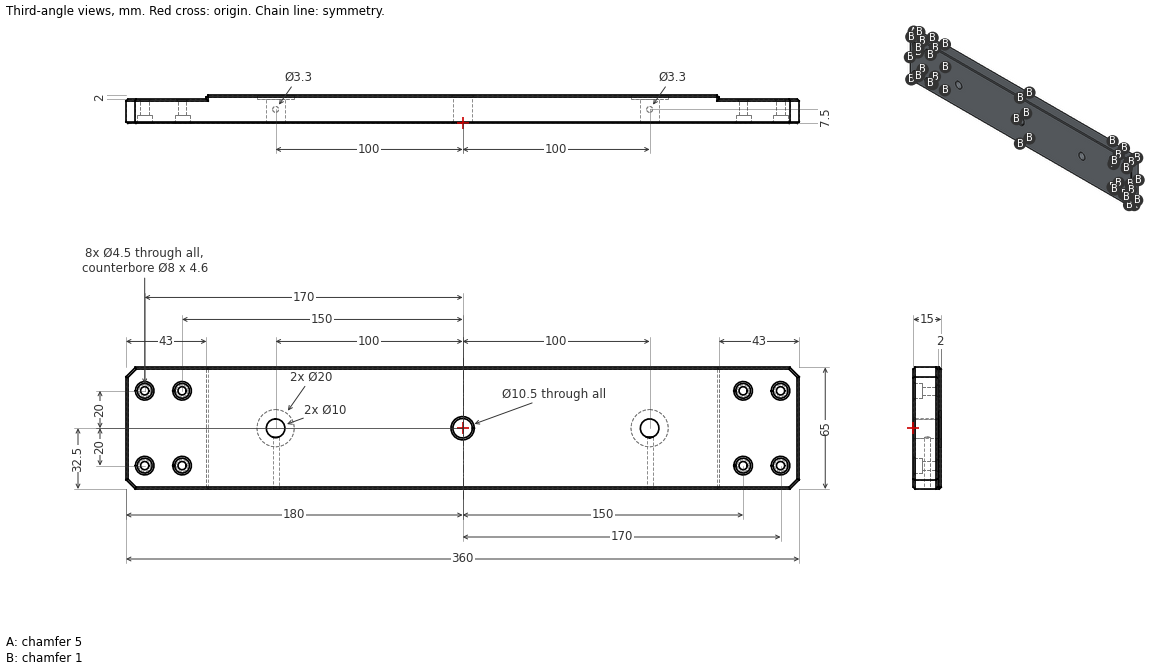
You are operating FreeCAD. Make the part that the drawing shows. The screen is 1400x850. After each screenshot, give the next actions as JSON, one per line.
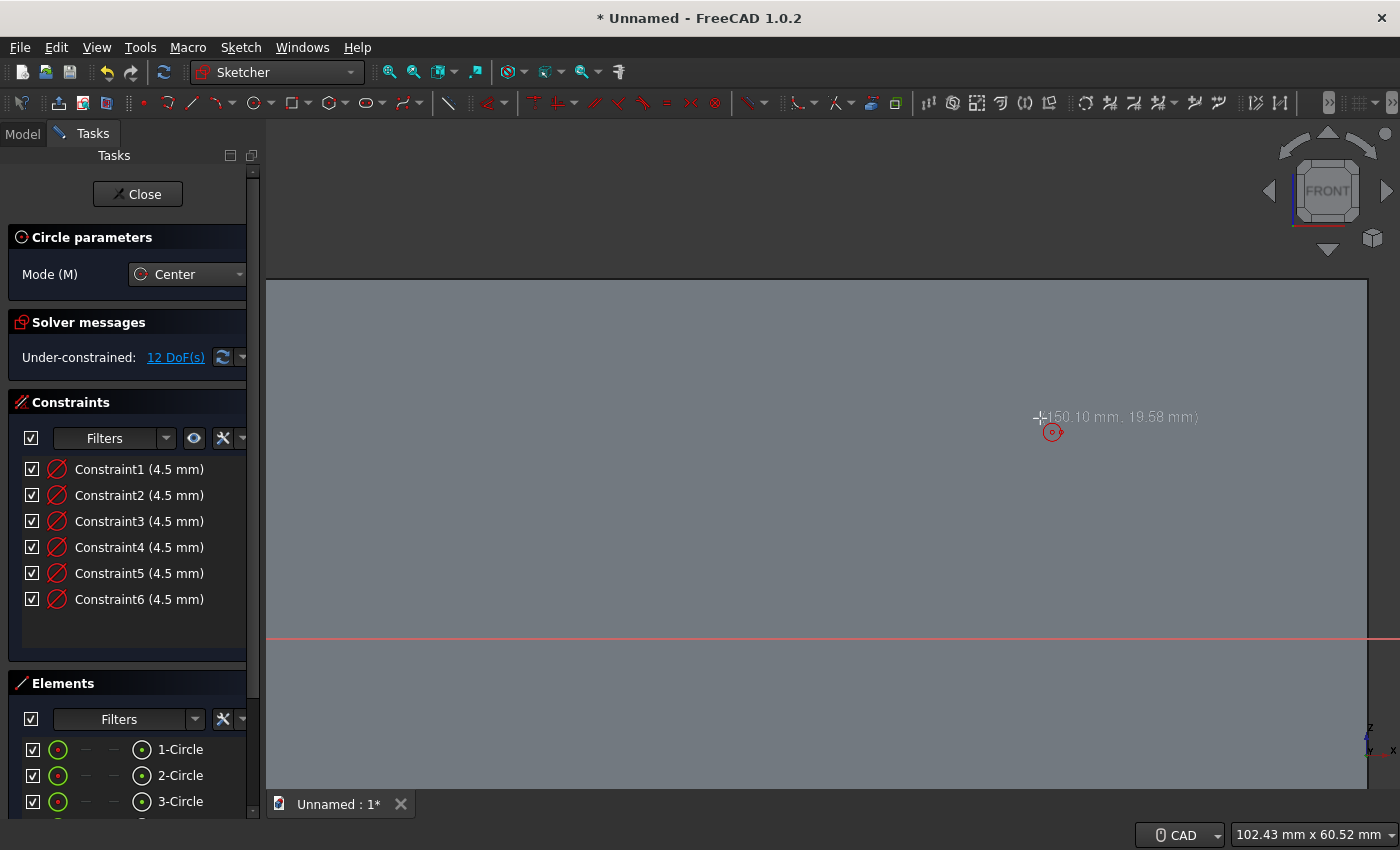
{"action": "scroll", "coordinate": [1040, 417], "scroll_direction": "down", "scroll_amount": 9}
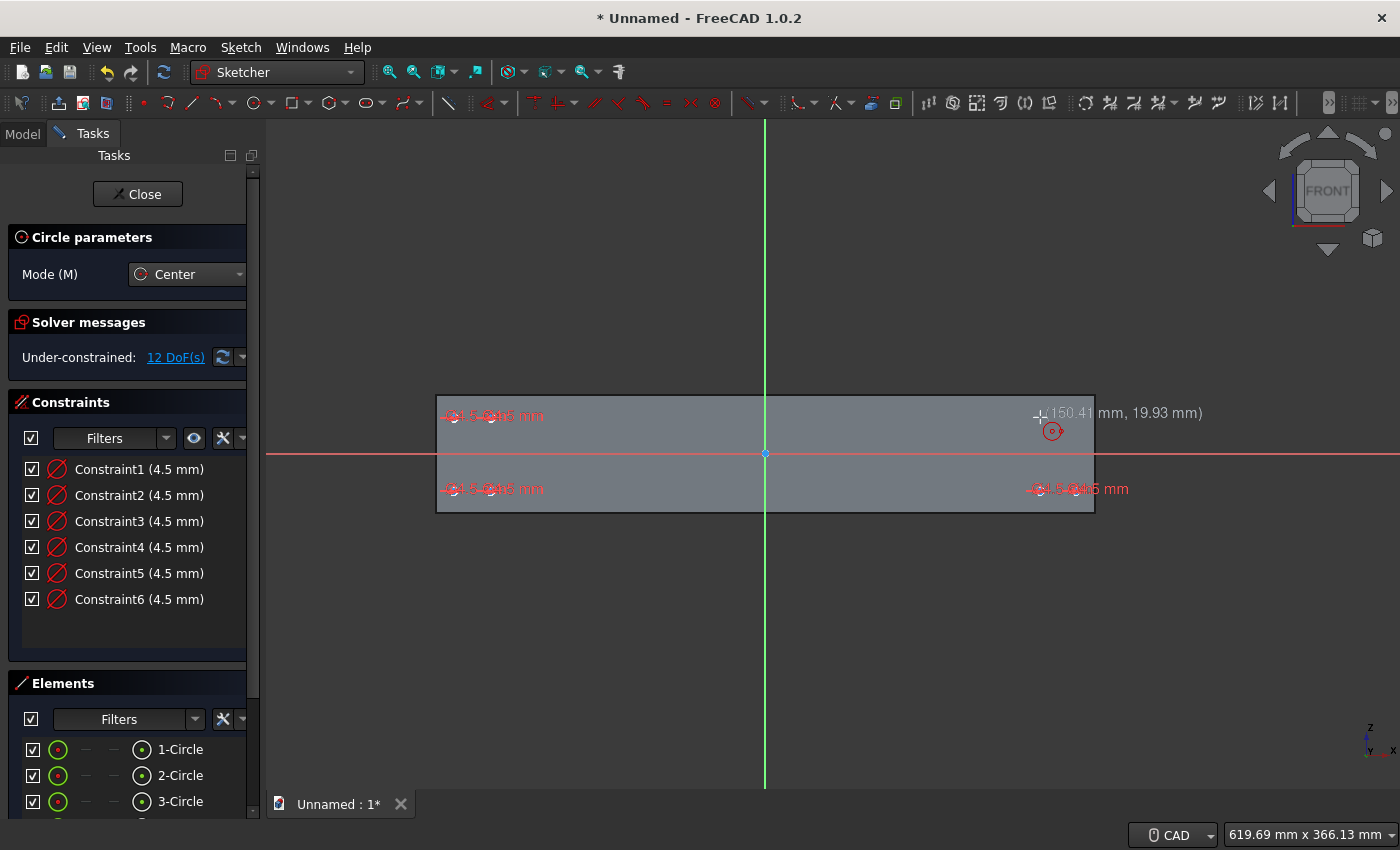
{"action": "left_click", "coordinate": [1040, 417]}
{"action": "mouse_move", "coordinate": [1043, 414]}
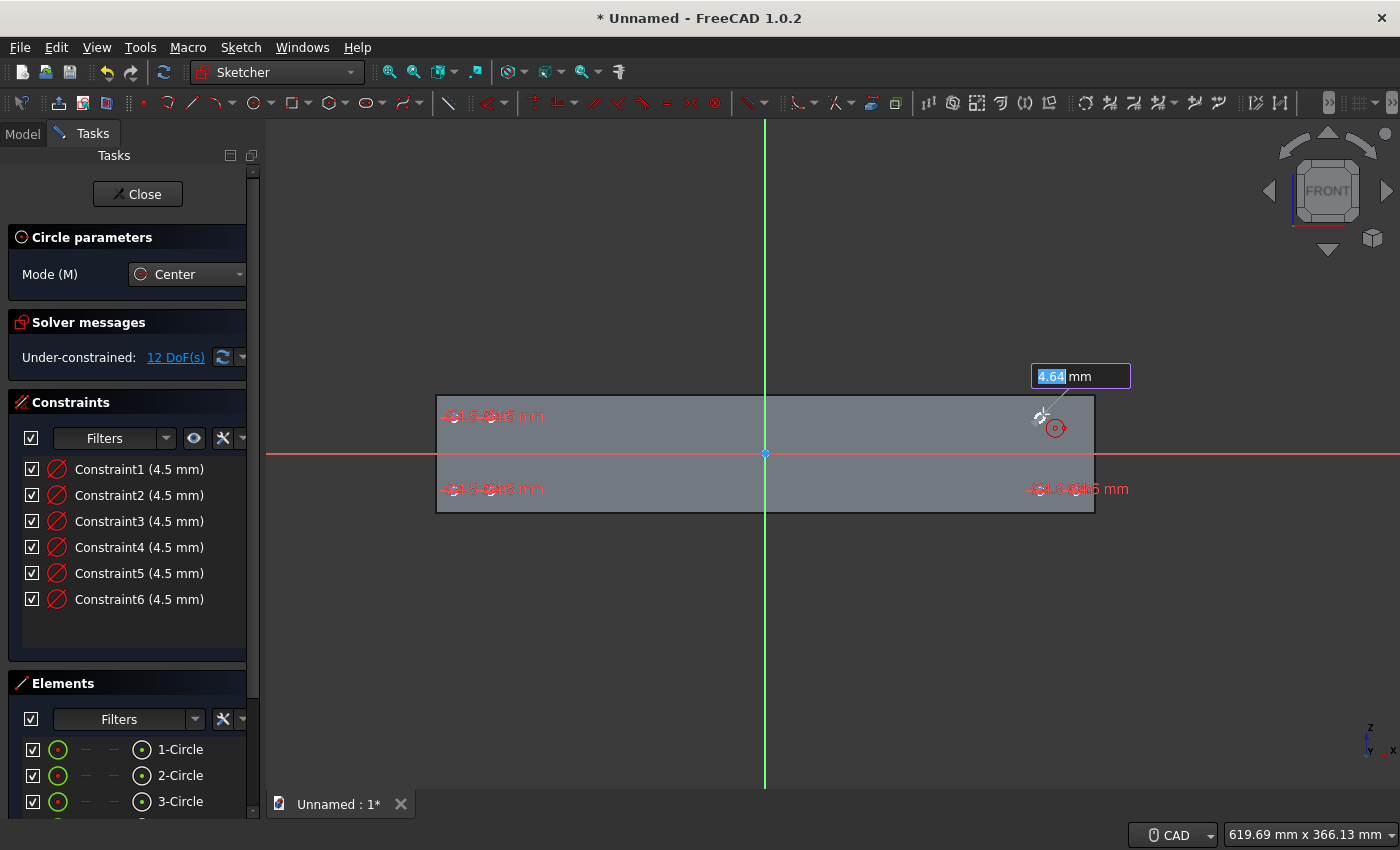
{"action": "type", "text": "4.5"}
{"action": "key", "text": "Return"}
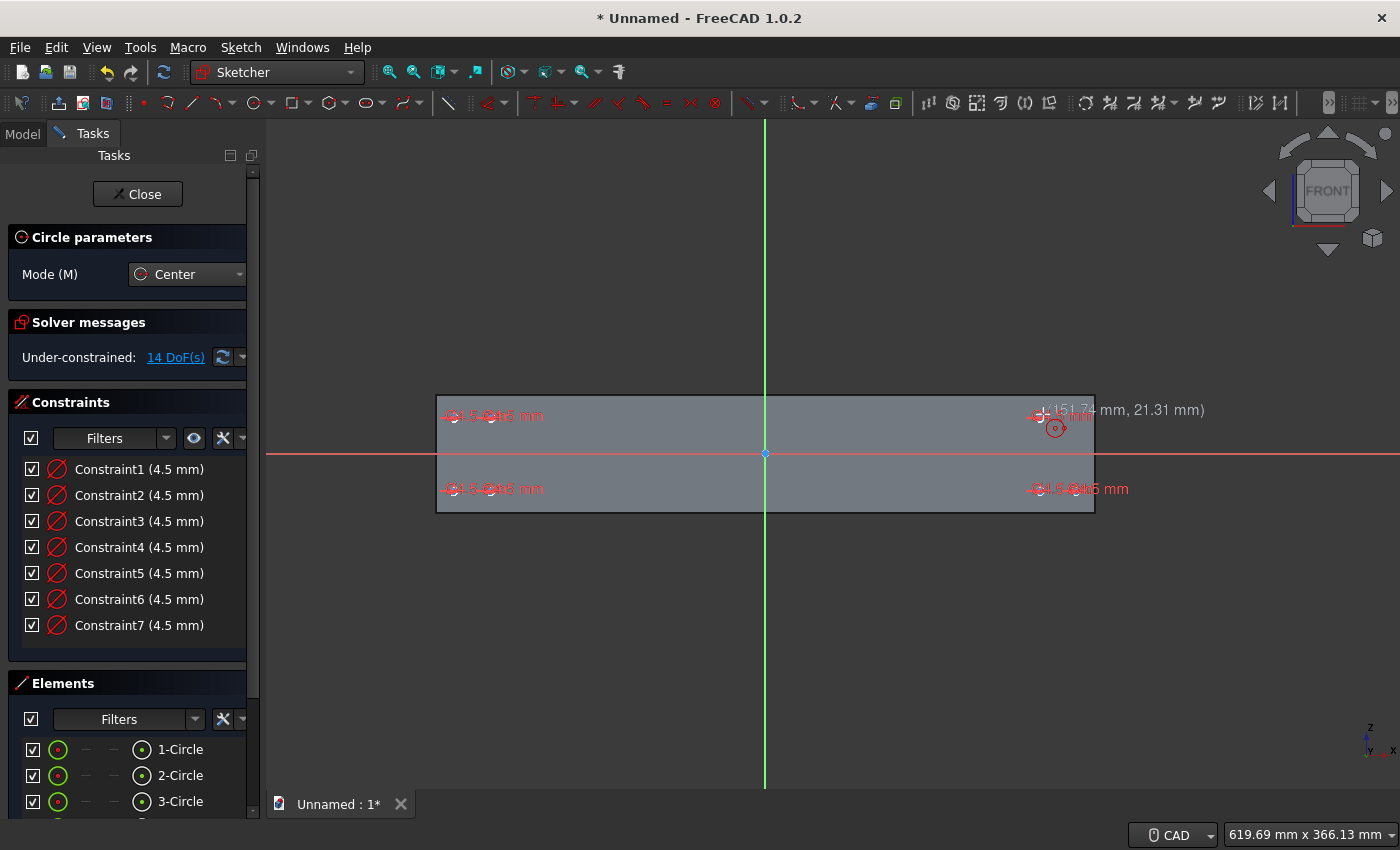
{"action": "scroll", "coordinate": [1076, 417], "scroll_direction": "up", "scroll_amount": 9}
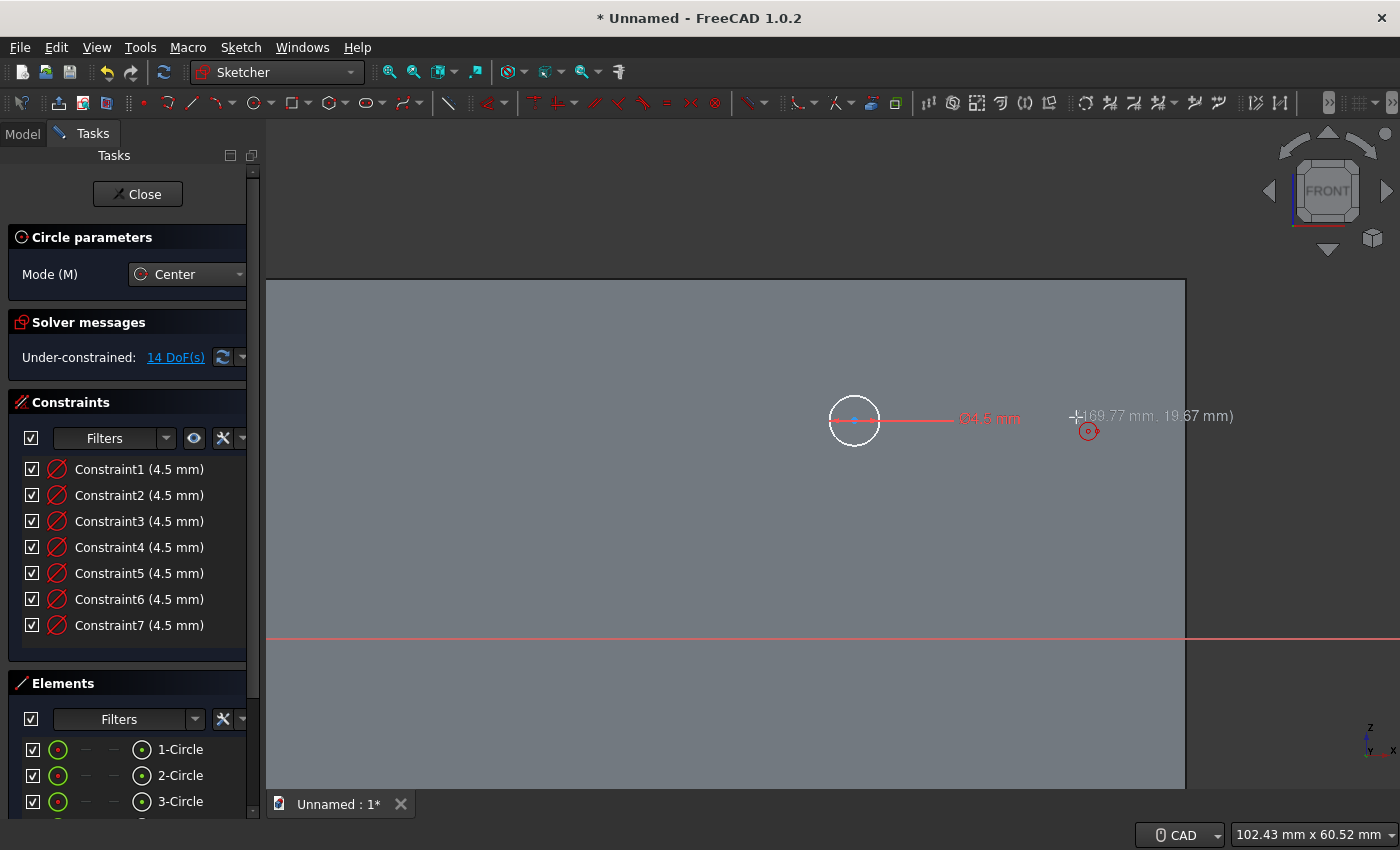
{"action": "scroll", "coordinate": [1076, 417], "scroll_direction": "down", "scroll_amount": 9}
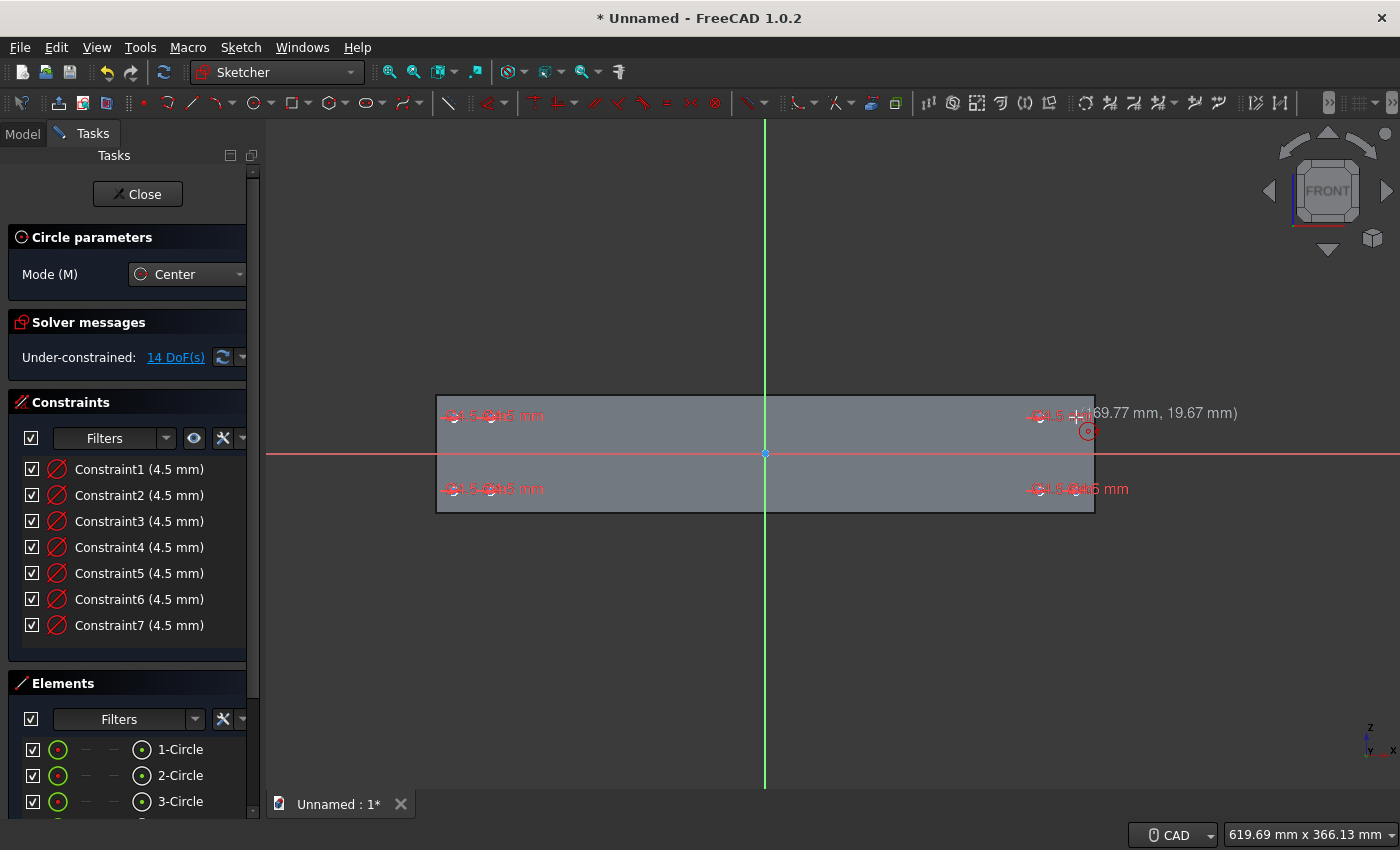
{"action": "left_click", "coordinate": [1076, 417]}
{"action": "mouse_move", "coordinate": [1079, 414]}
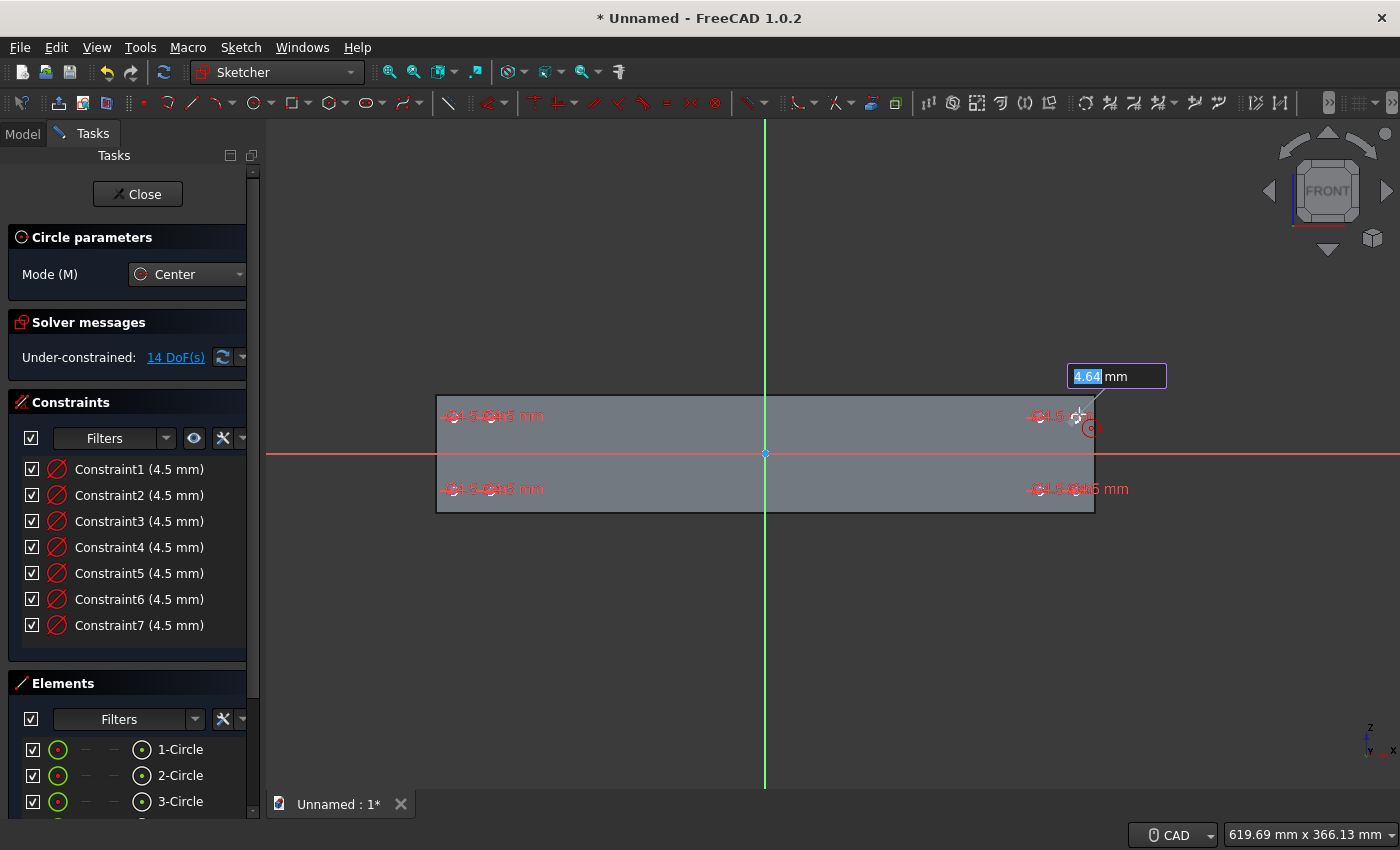
{"action": "type", "text": "4.5"}
{"action": "key", "text": "Return"}
{"action": "key", "text": "Escape"}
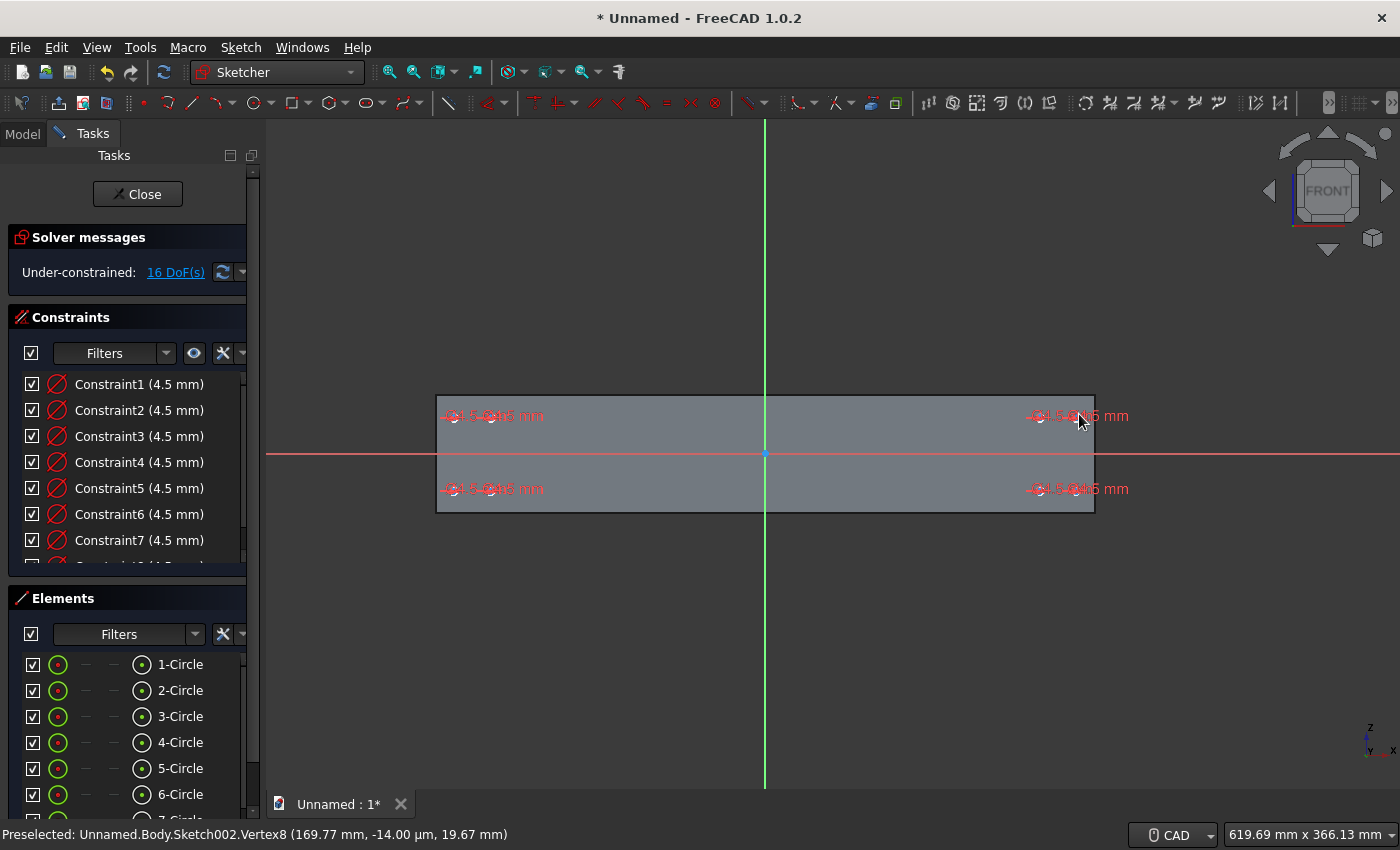
{"action": "left_click", "coordinate": [454, 418]}